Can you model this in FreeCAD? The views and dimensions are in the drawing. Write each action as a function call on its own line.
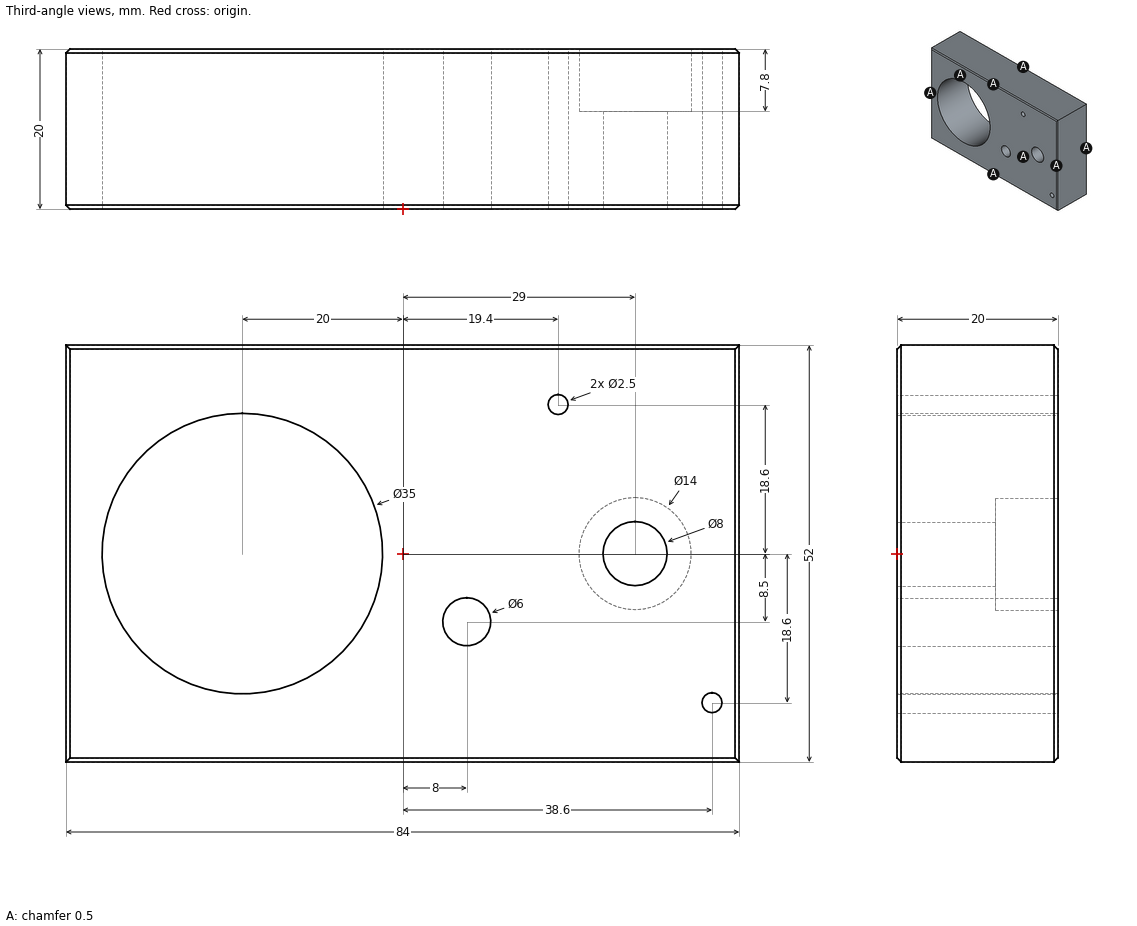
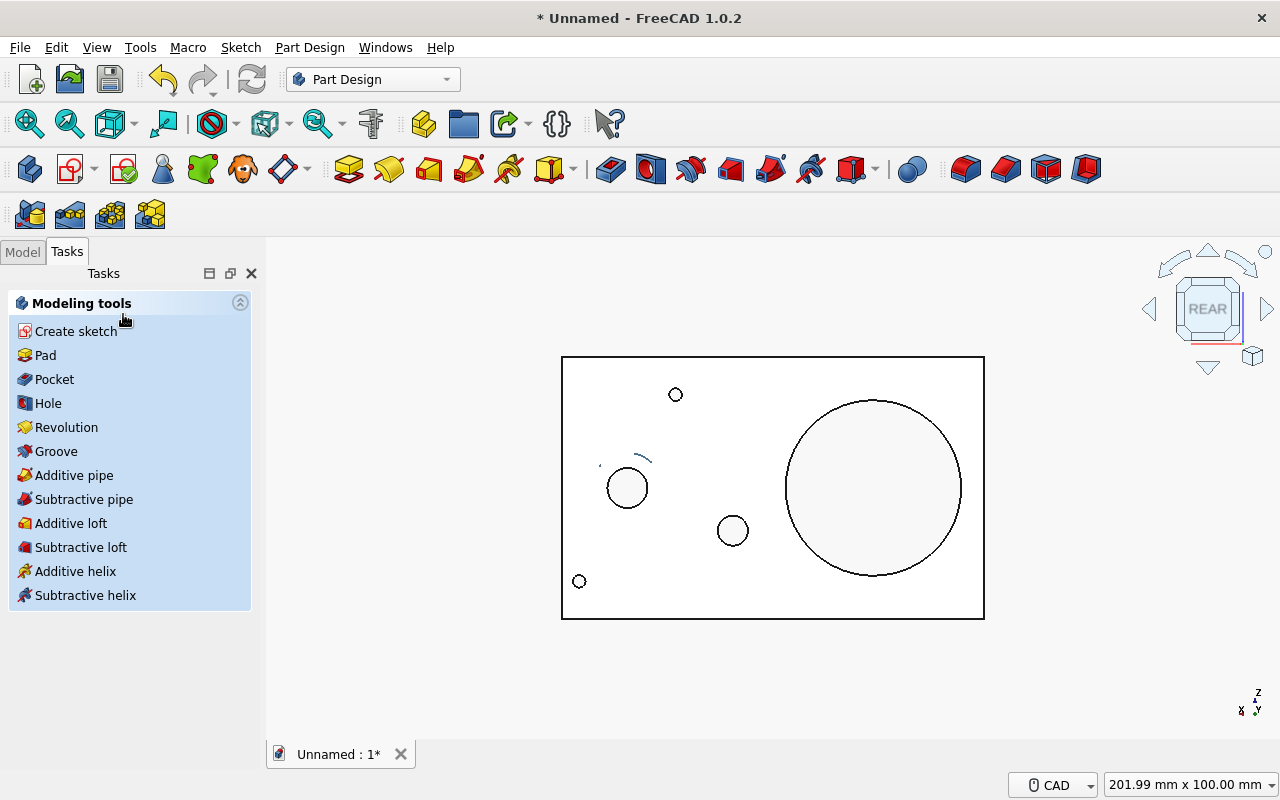
click(612, 170)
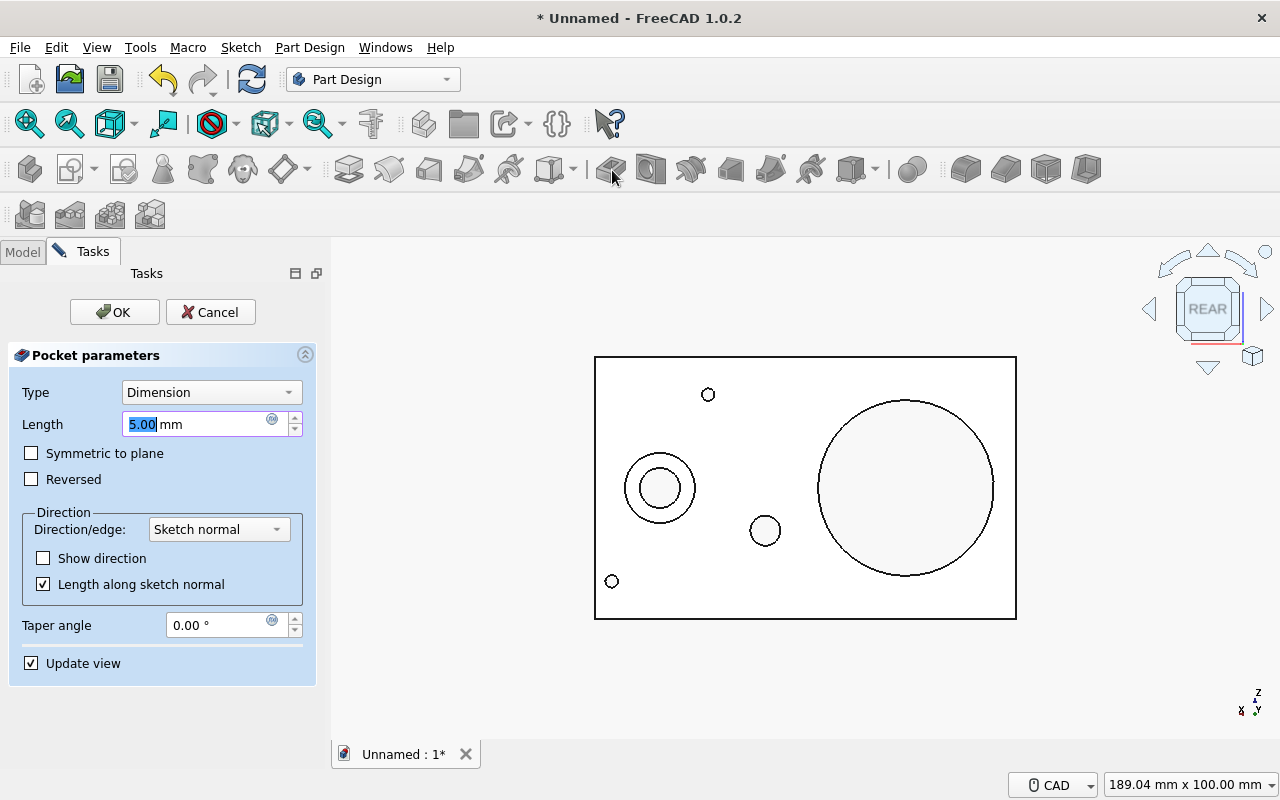
text(7.8)
key(Tab)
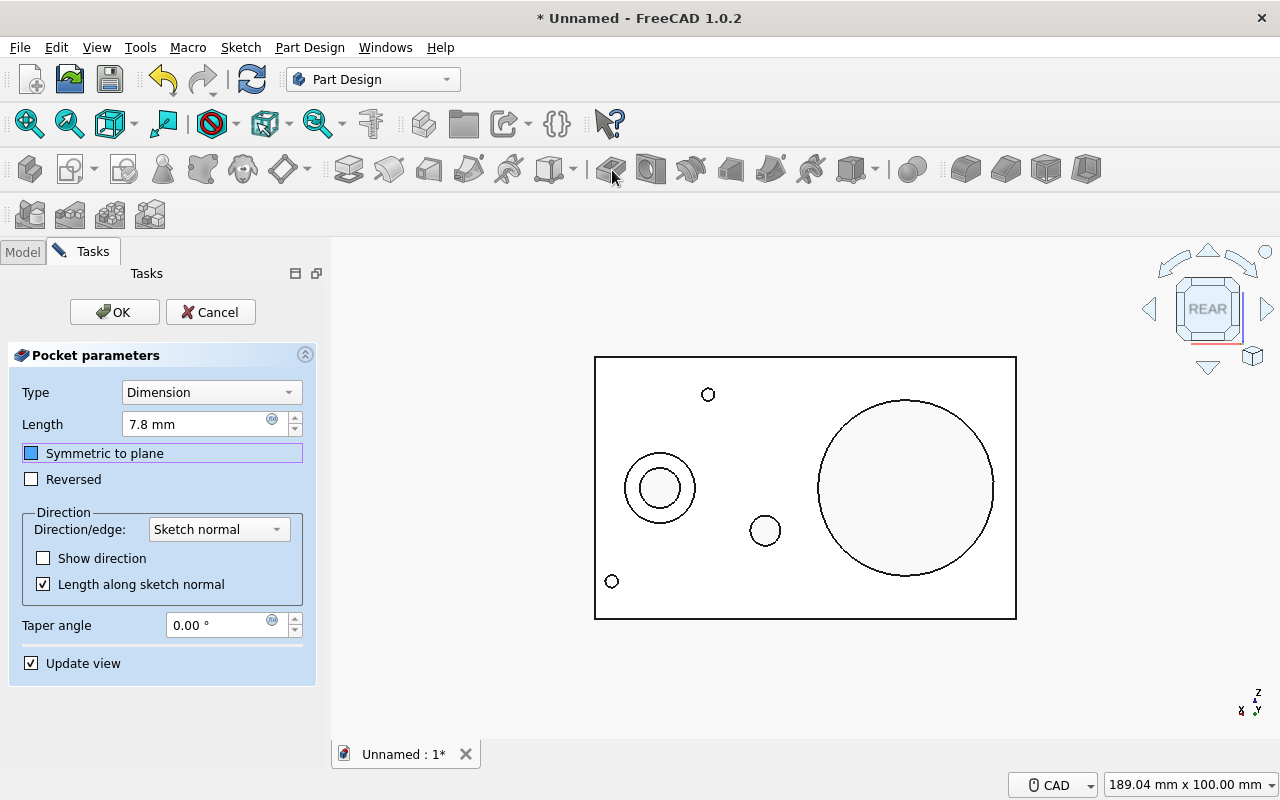
click(115, 312)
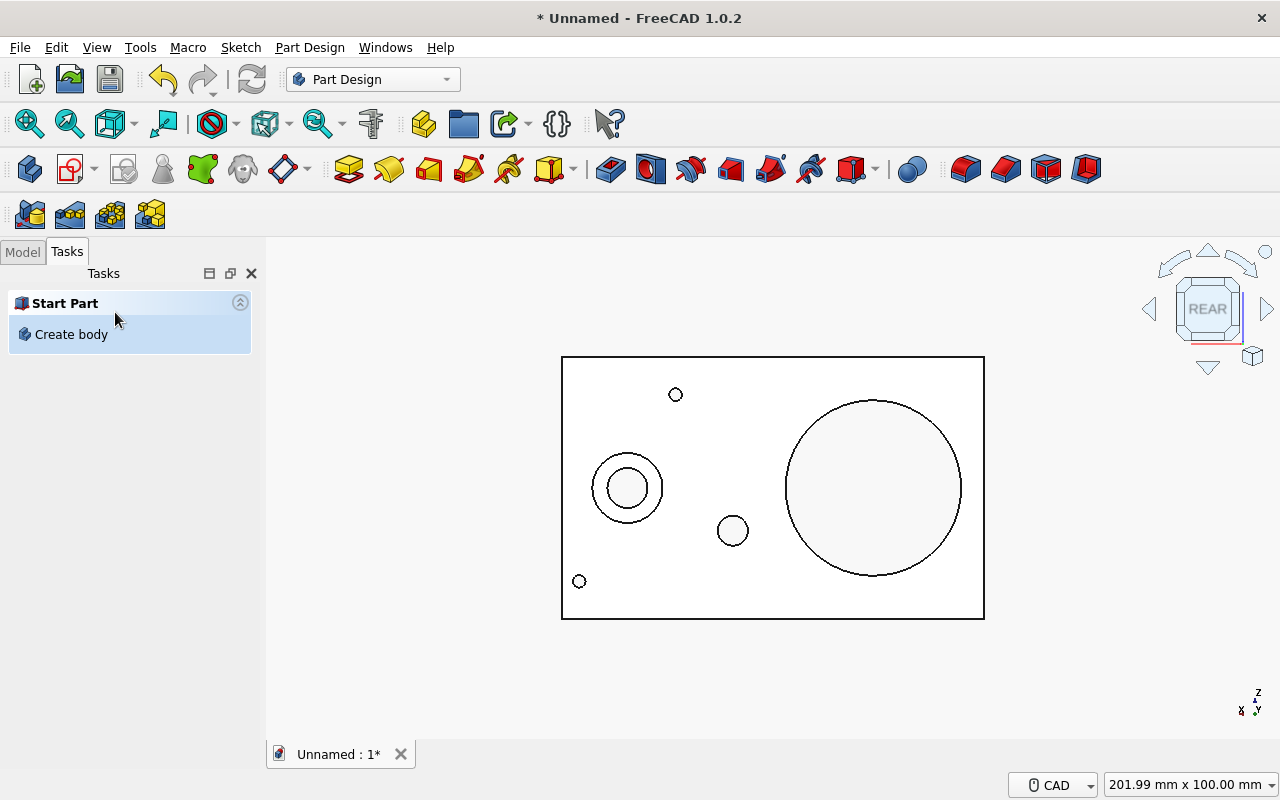
click(984, 487)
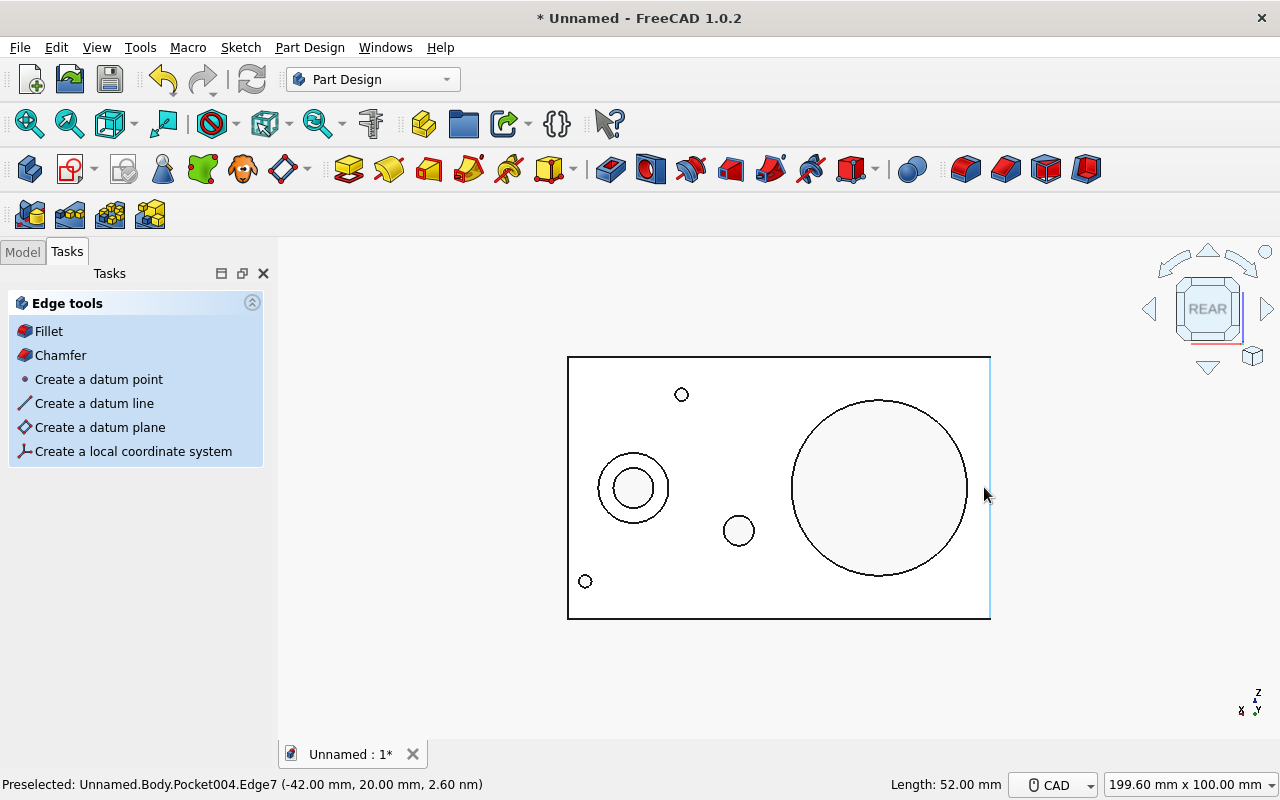
click(779, 618, ctrl)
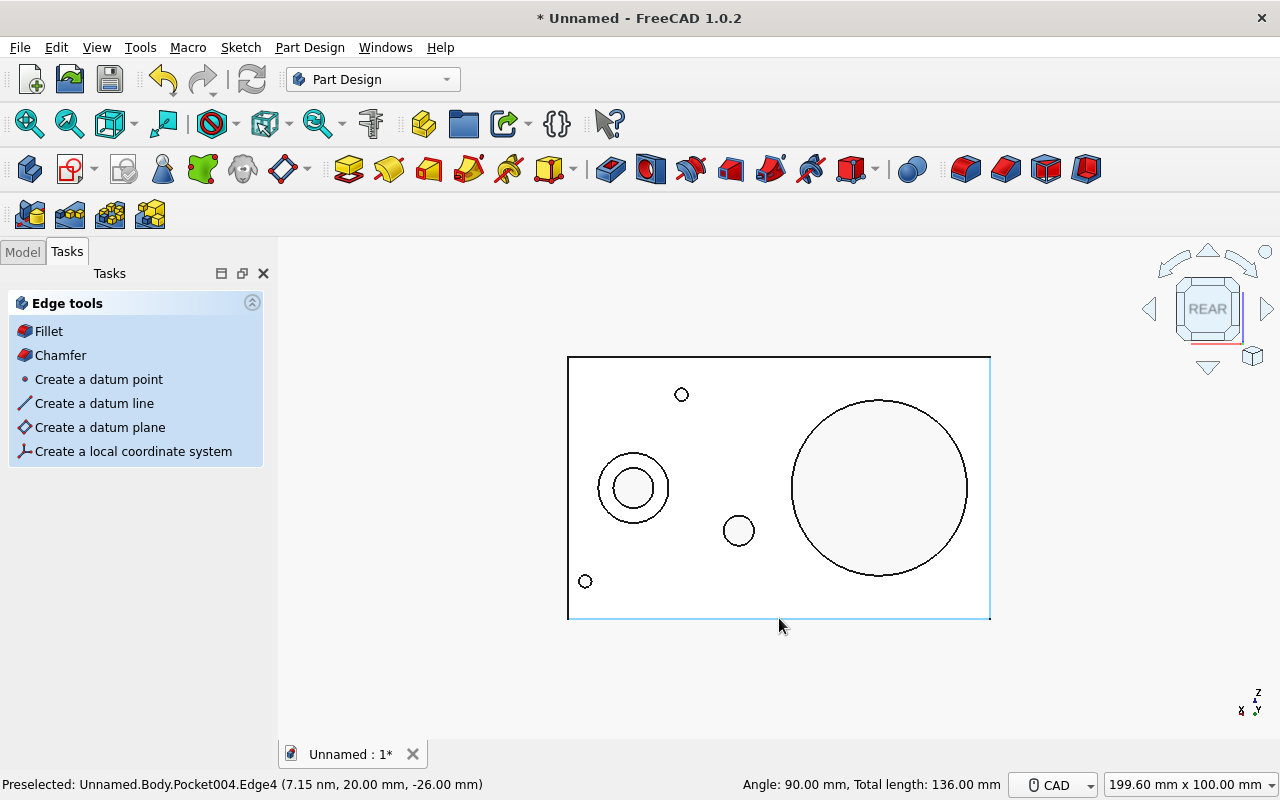
key(0)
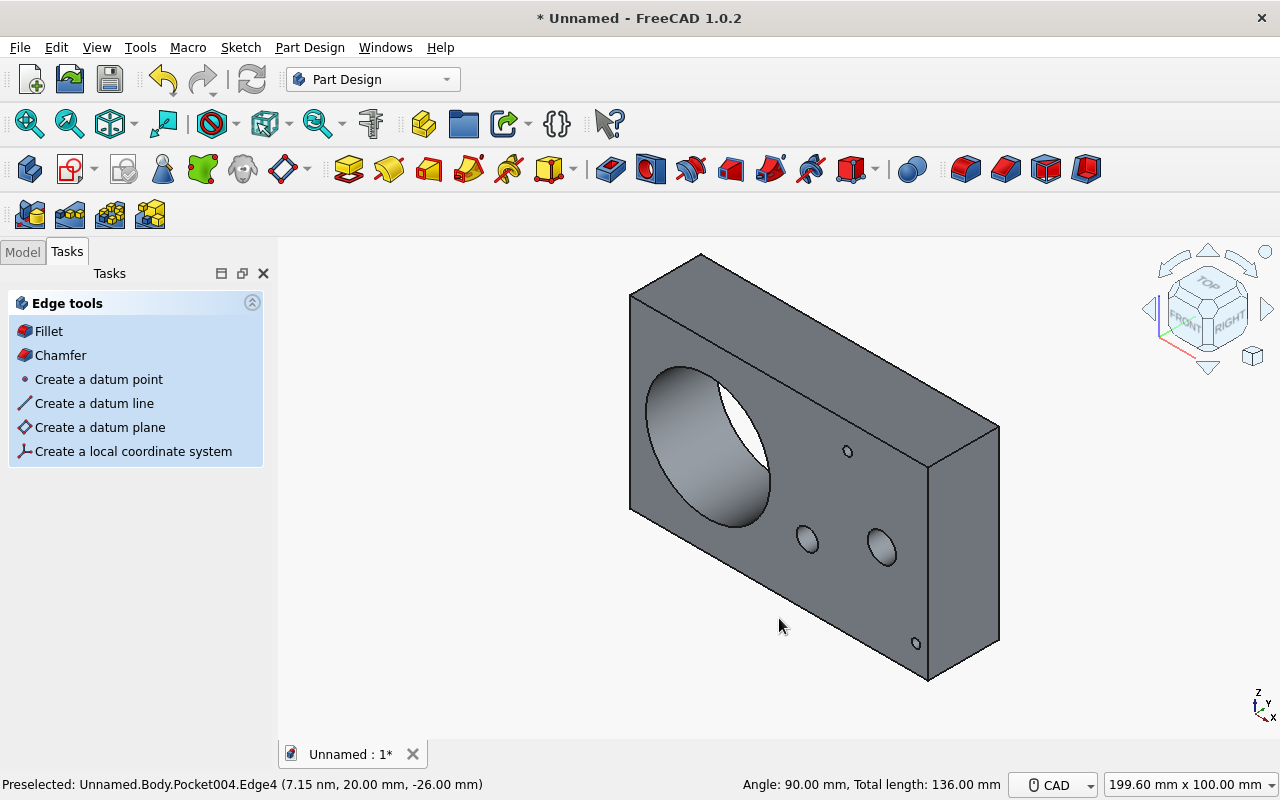
click(779, 380, ctrl)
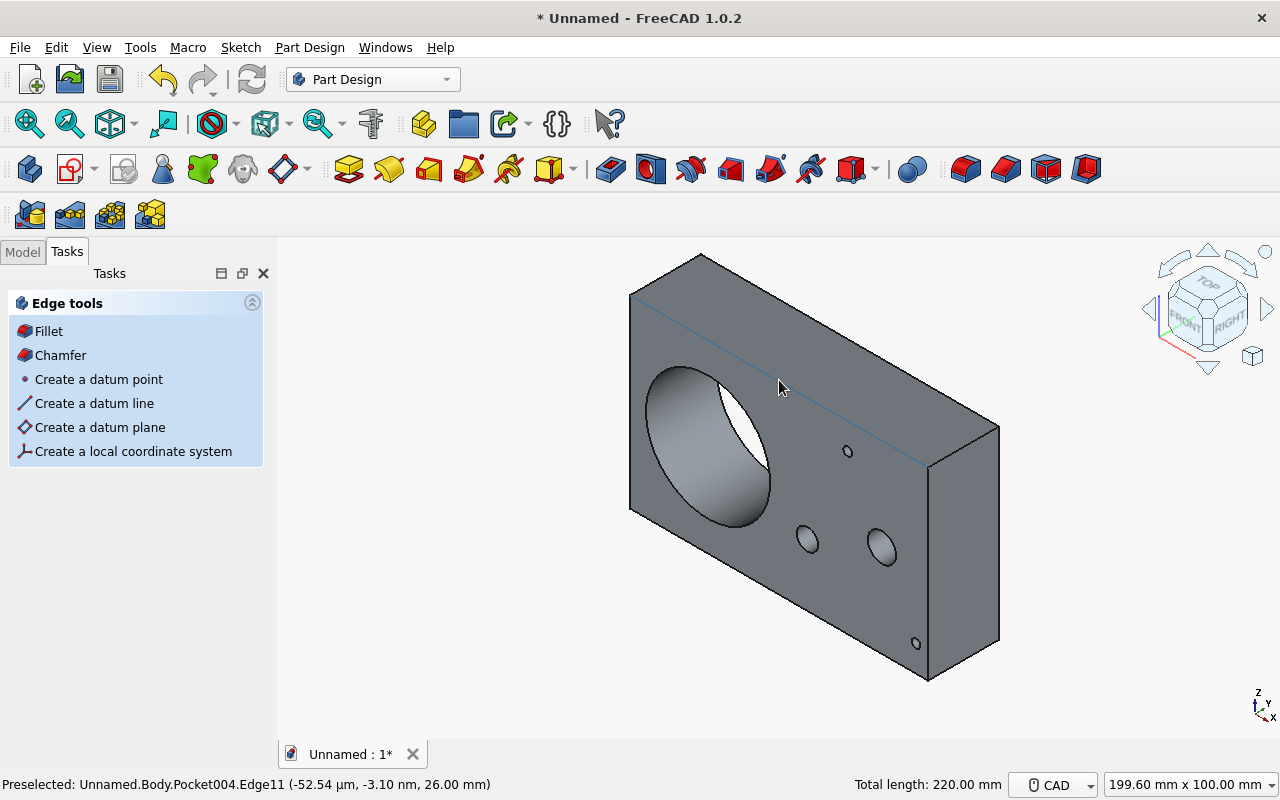
click(928, 573, ctrl)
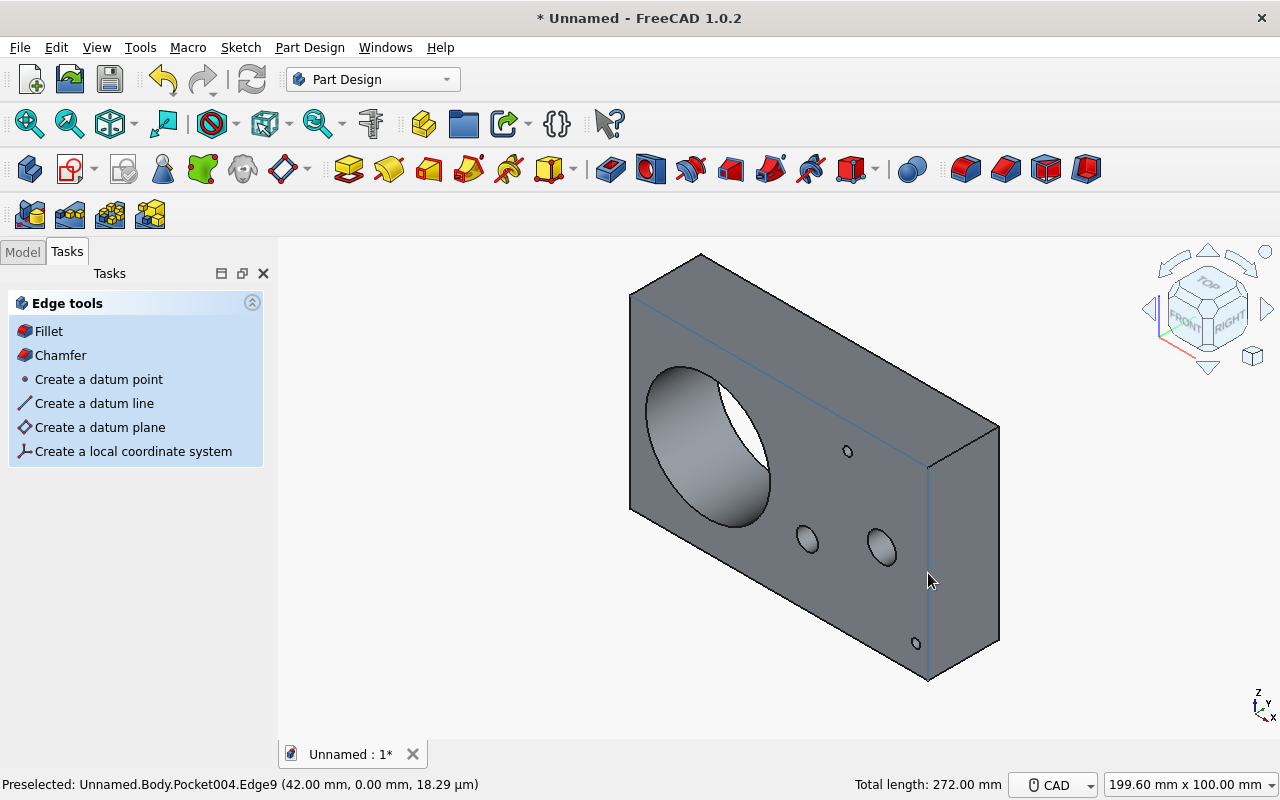
key(2)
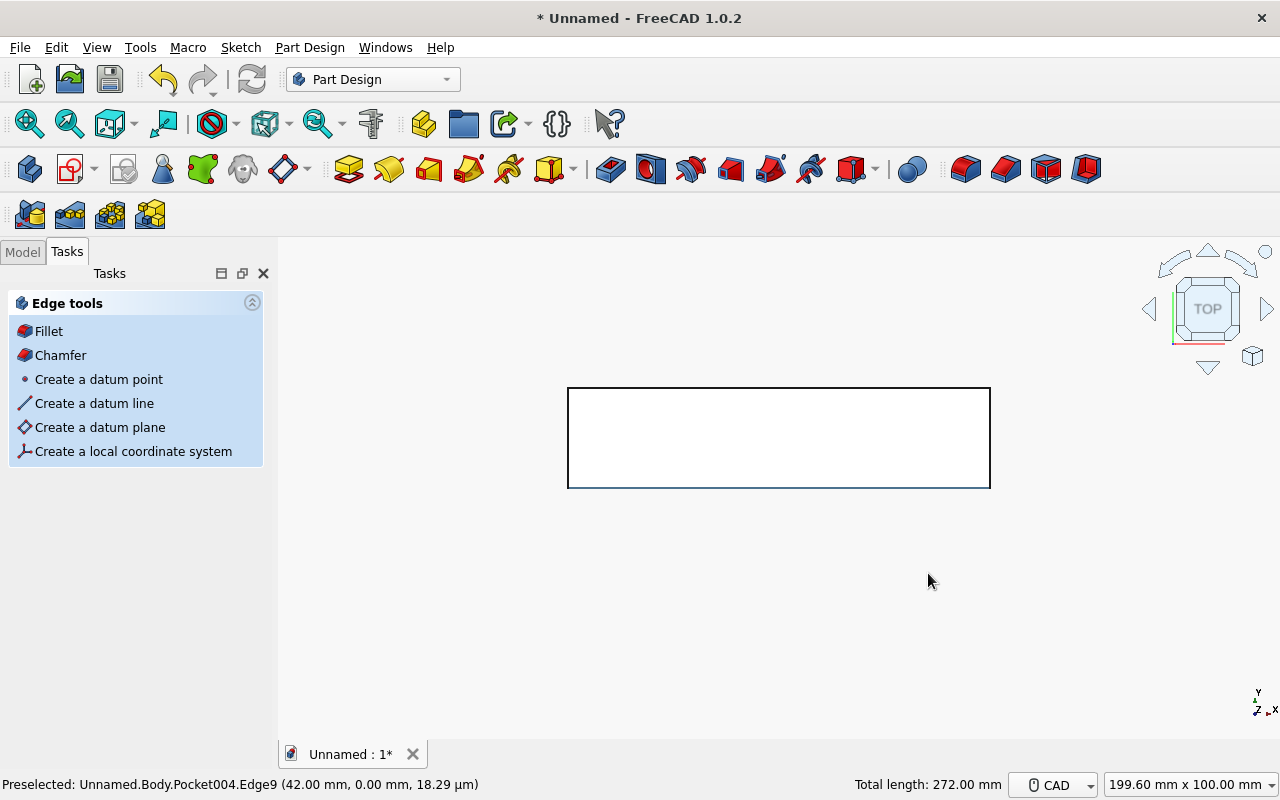
click(30, 124)